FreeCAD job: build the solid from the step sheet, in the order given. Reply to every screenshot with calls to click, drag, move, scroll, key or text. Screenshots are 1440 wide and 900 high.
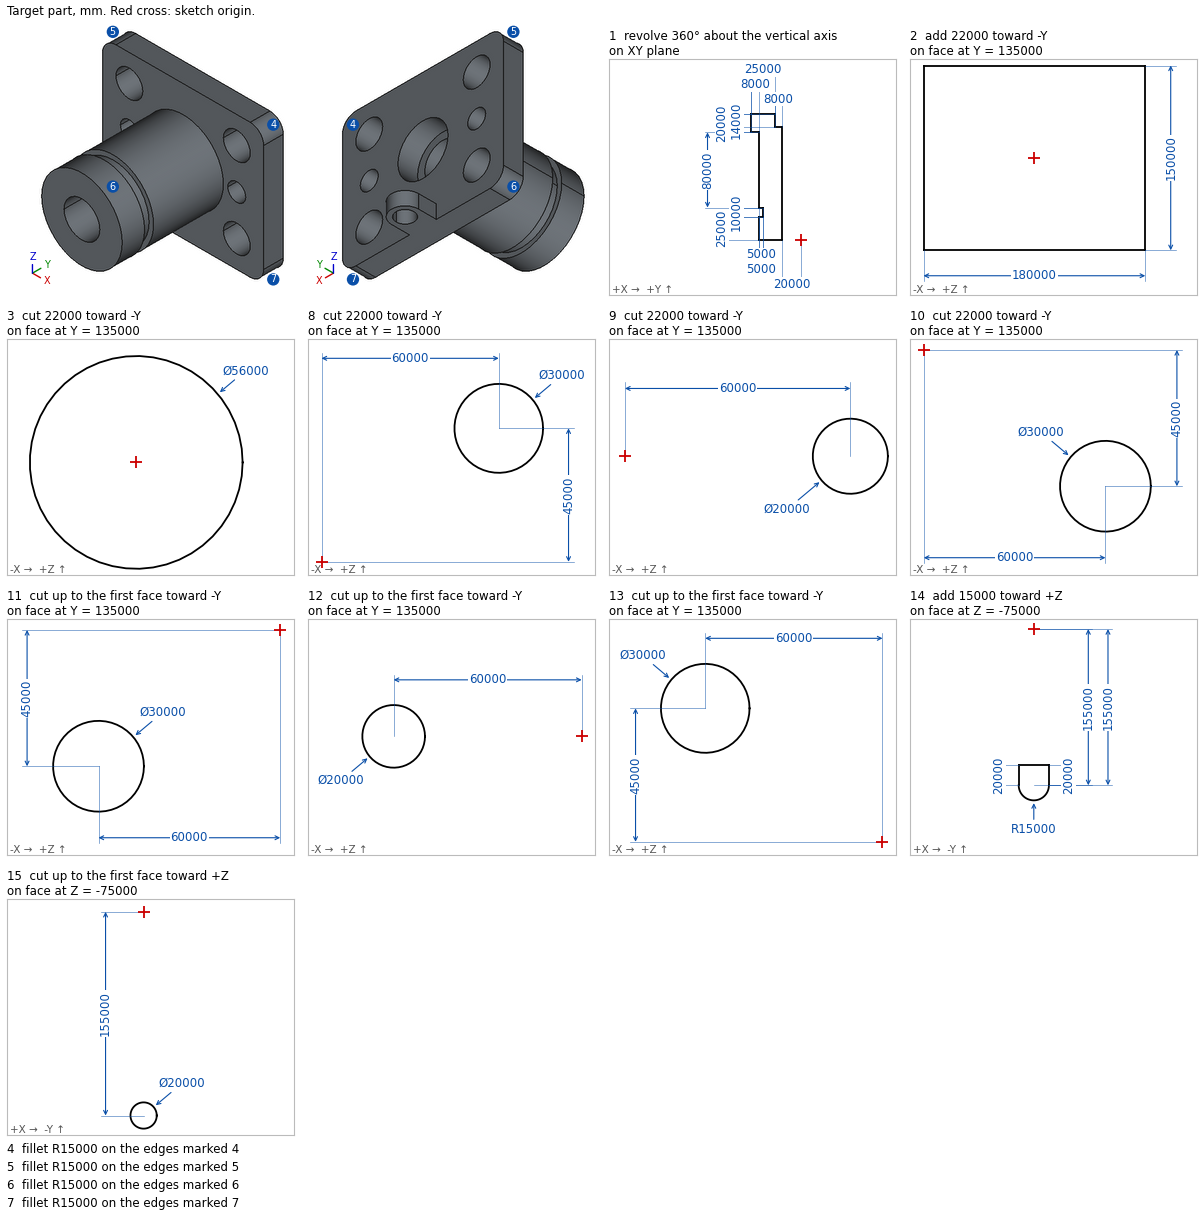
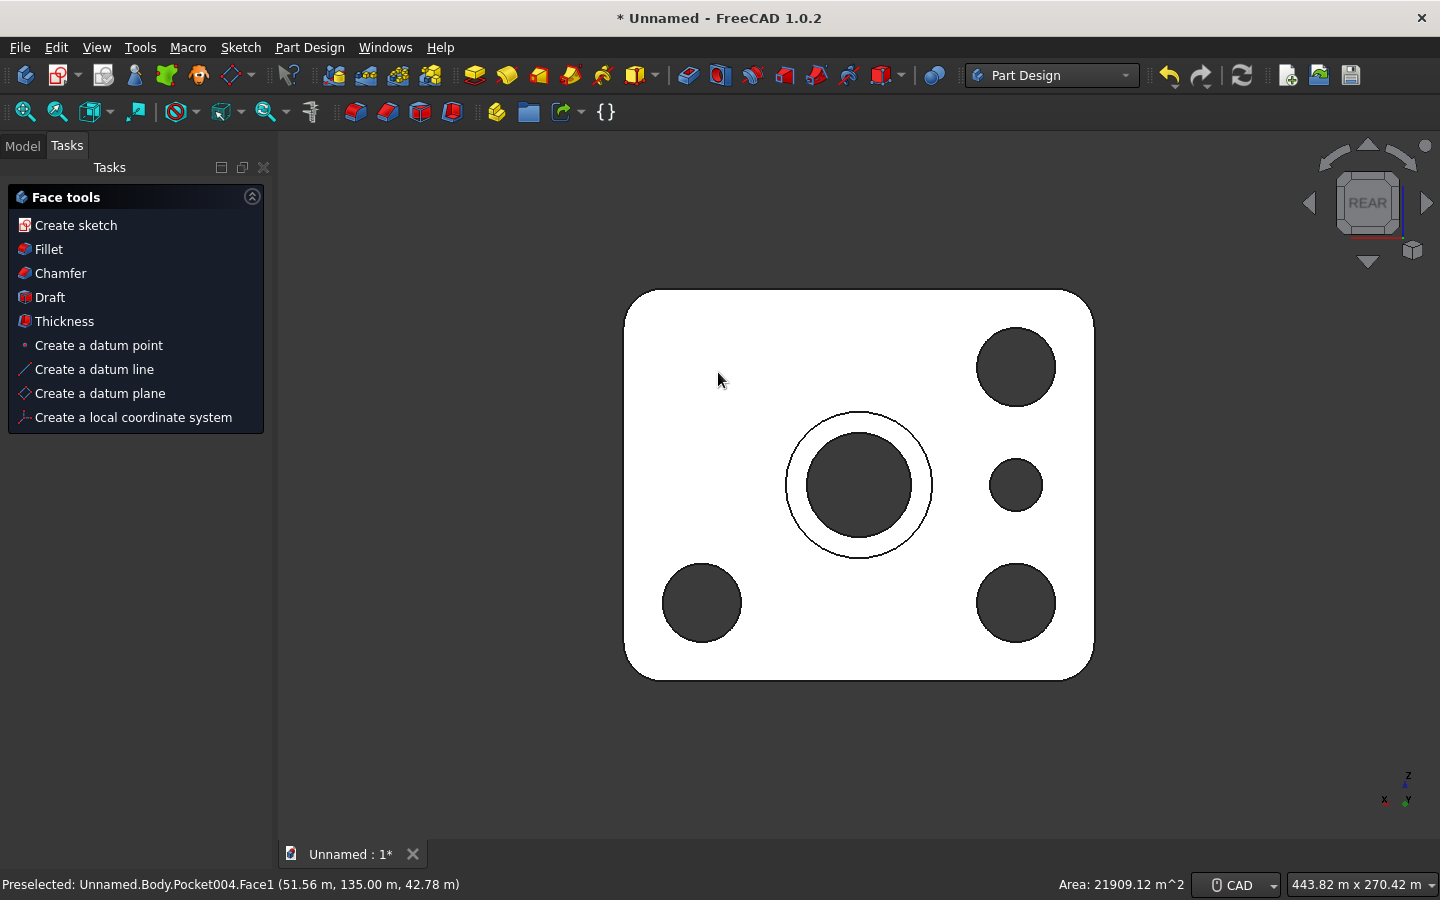
click(58, 76)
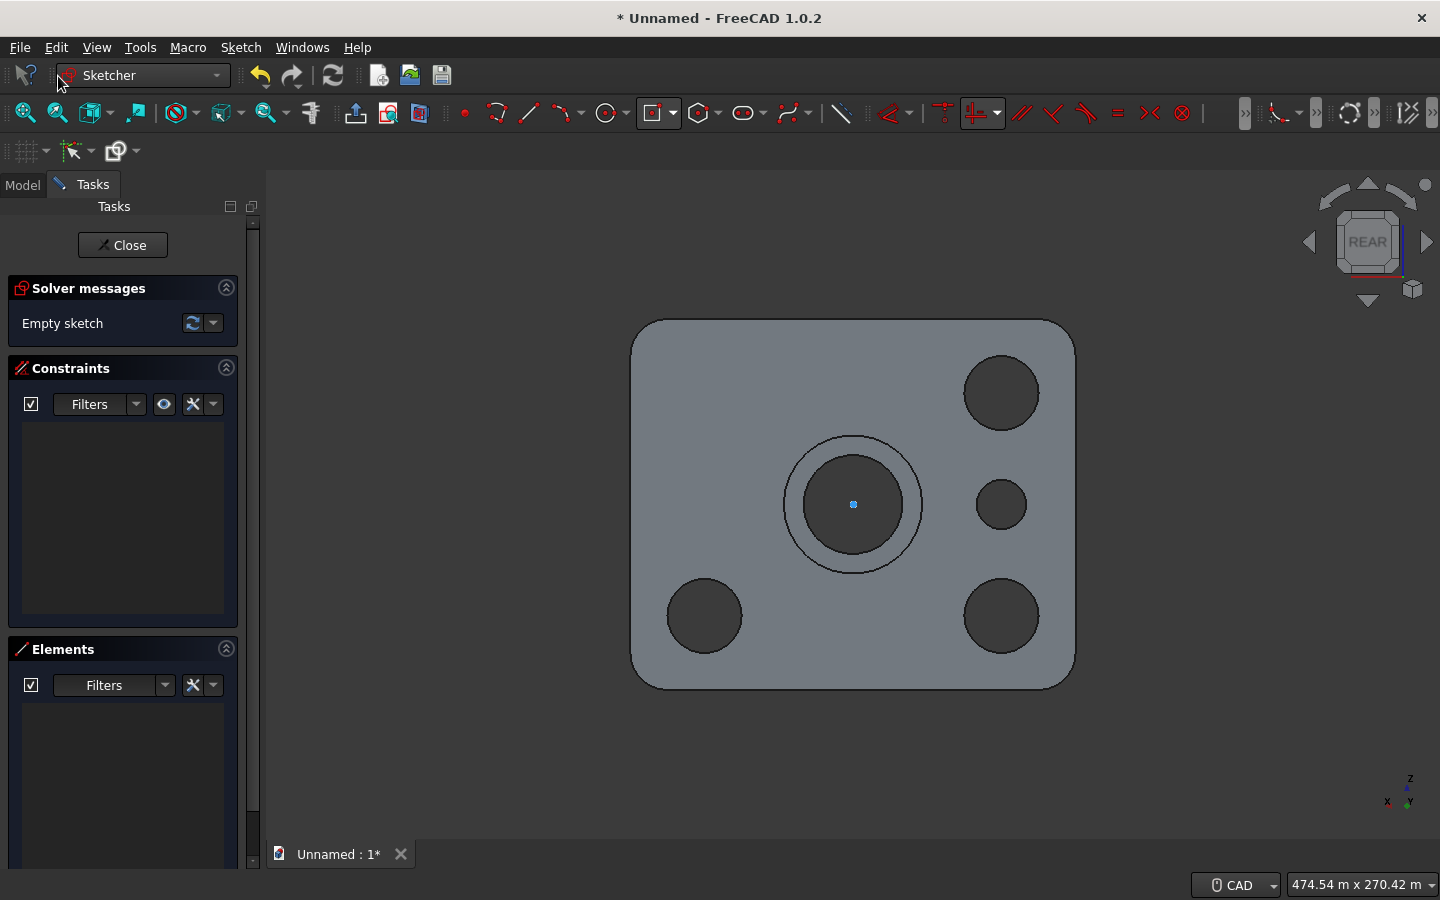
scroll(695, 504, up, 11)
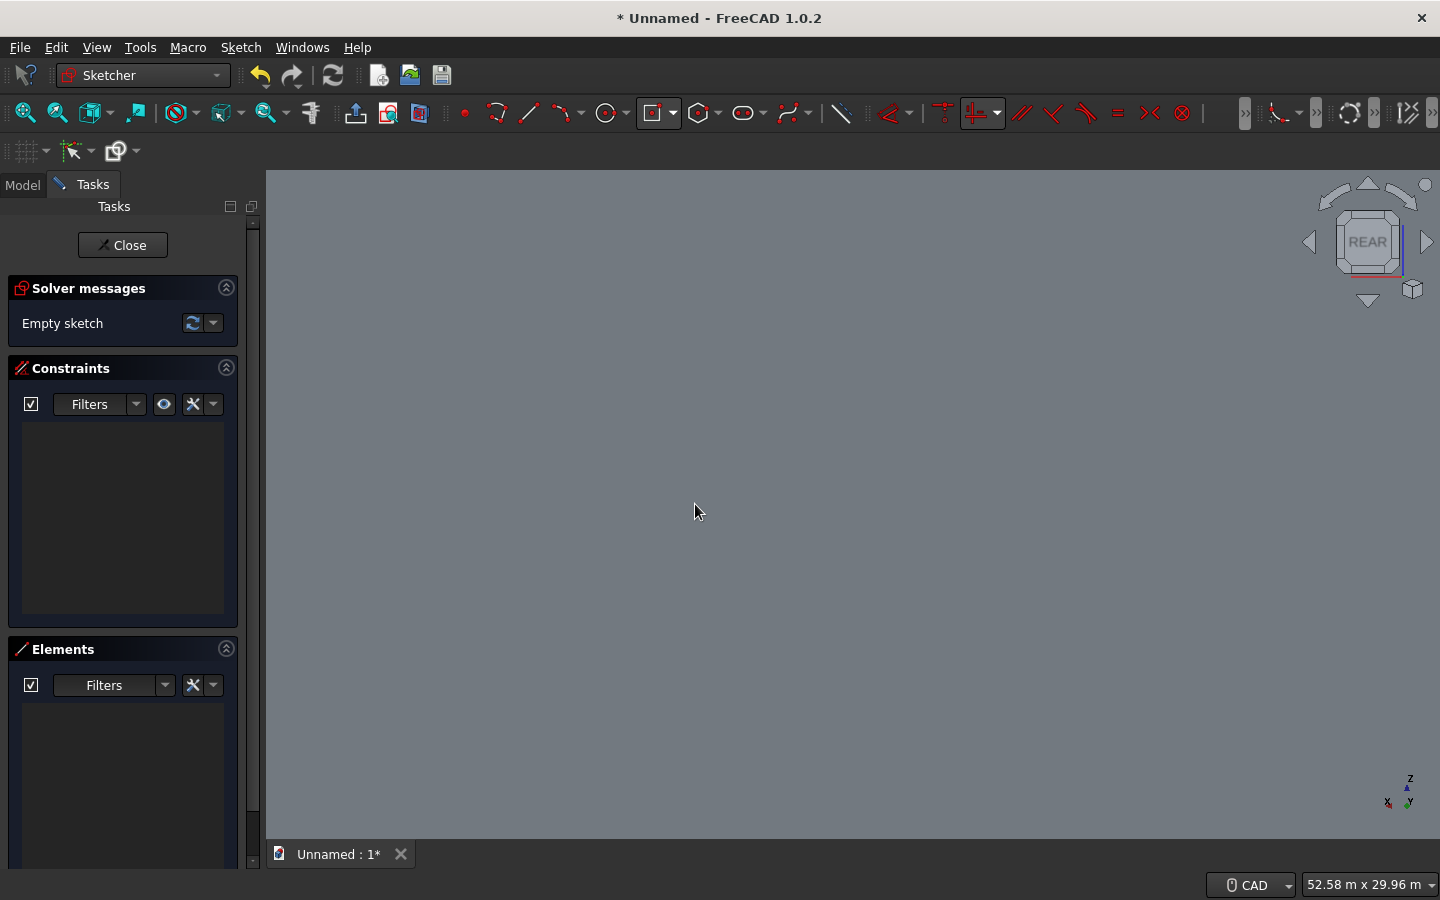
key(g)
key(c)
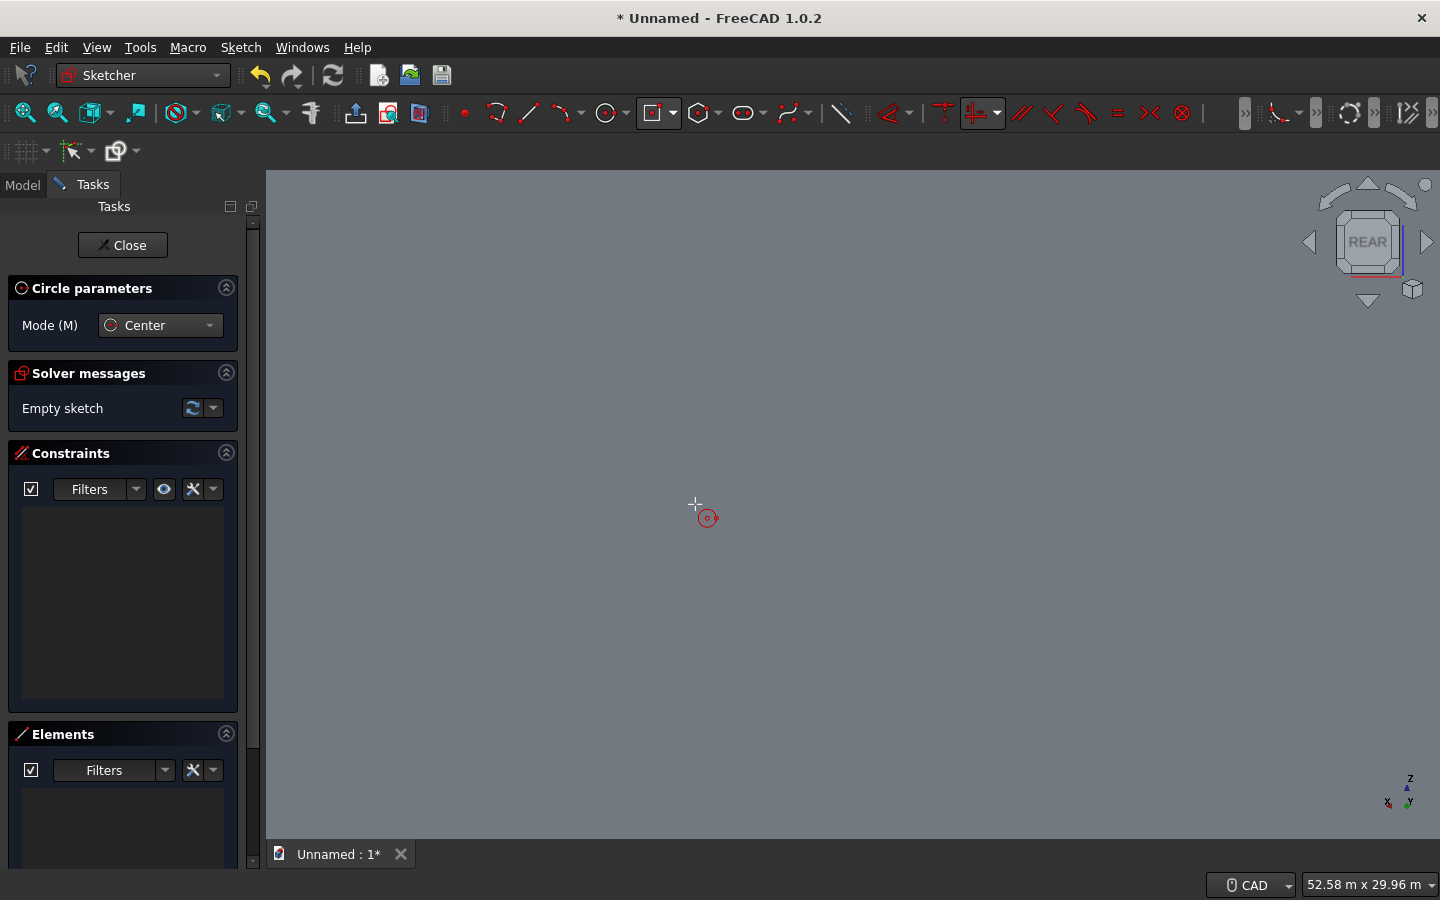
click(778, 504)
click(936, 347)
key(Escape)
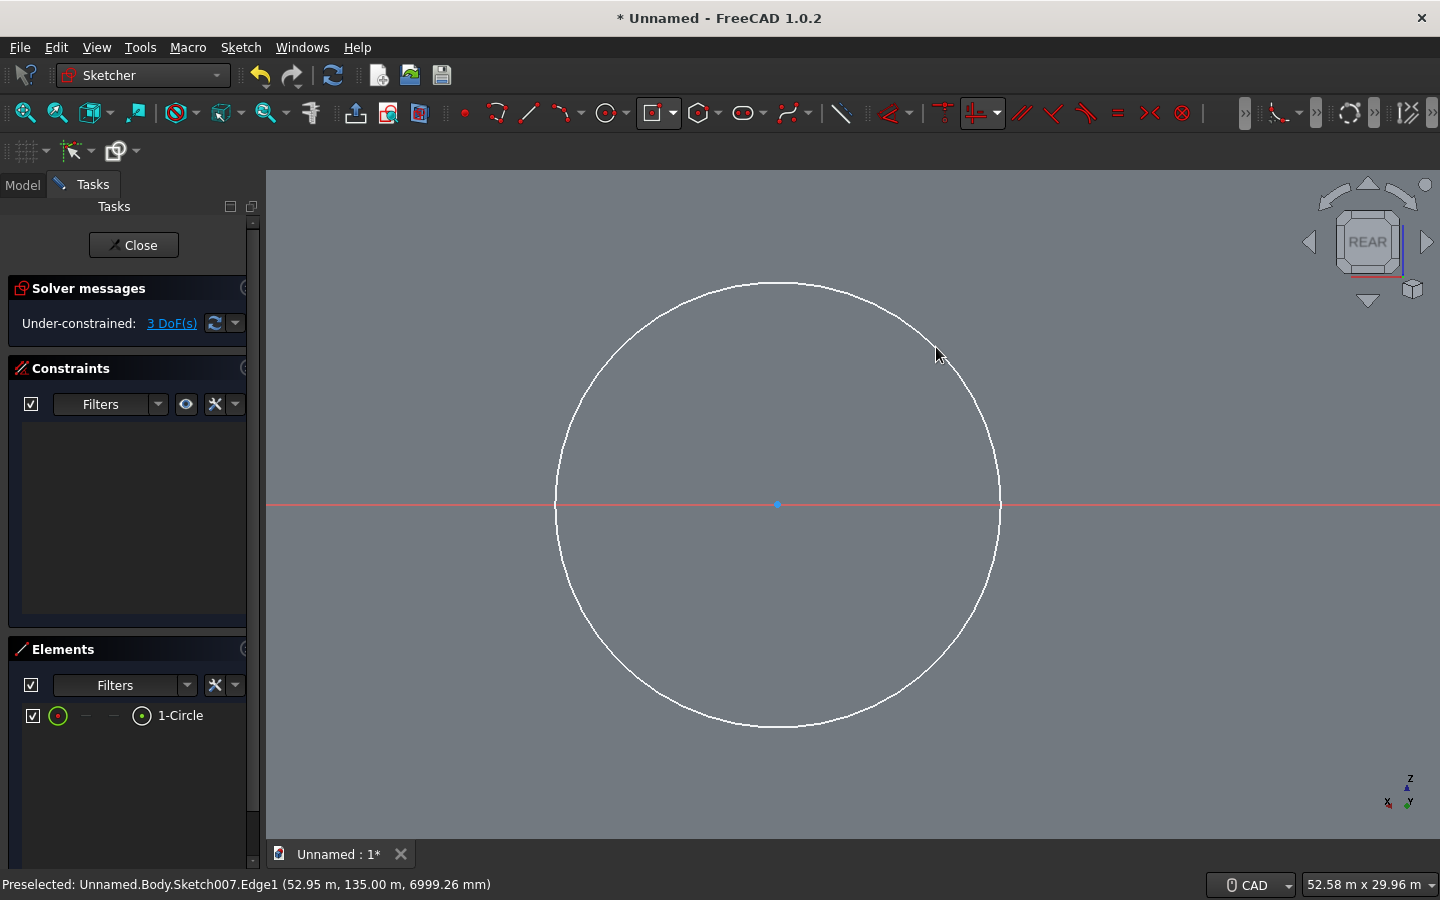
click(778, 505)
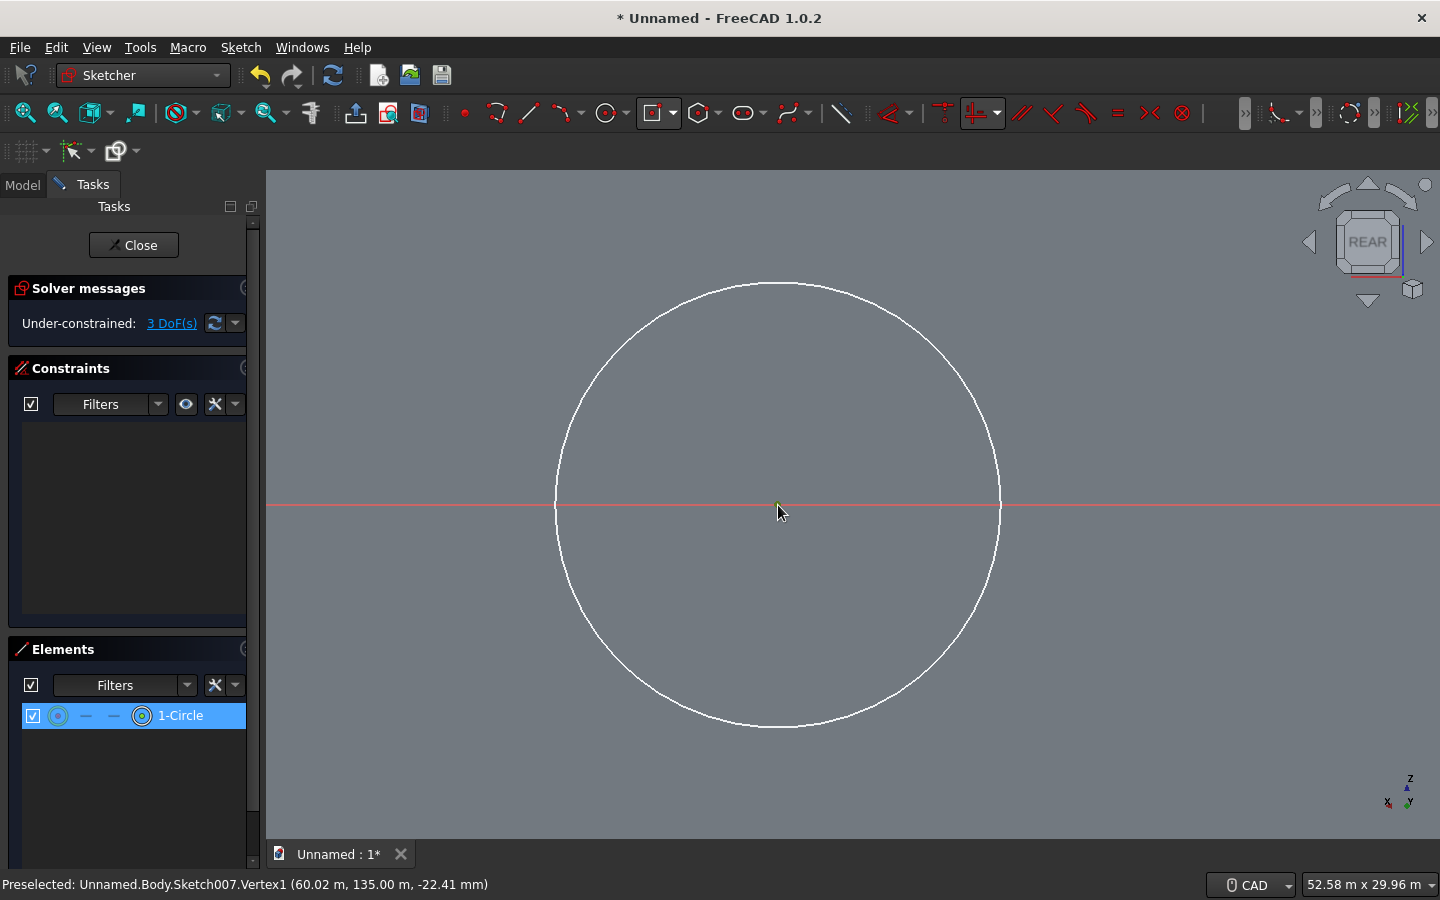
click(364, 504)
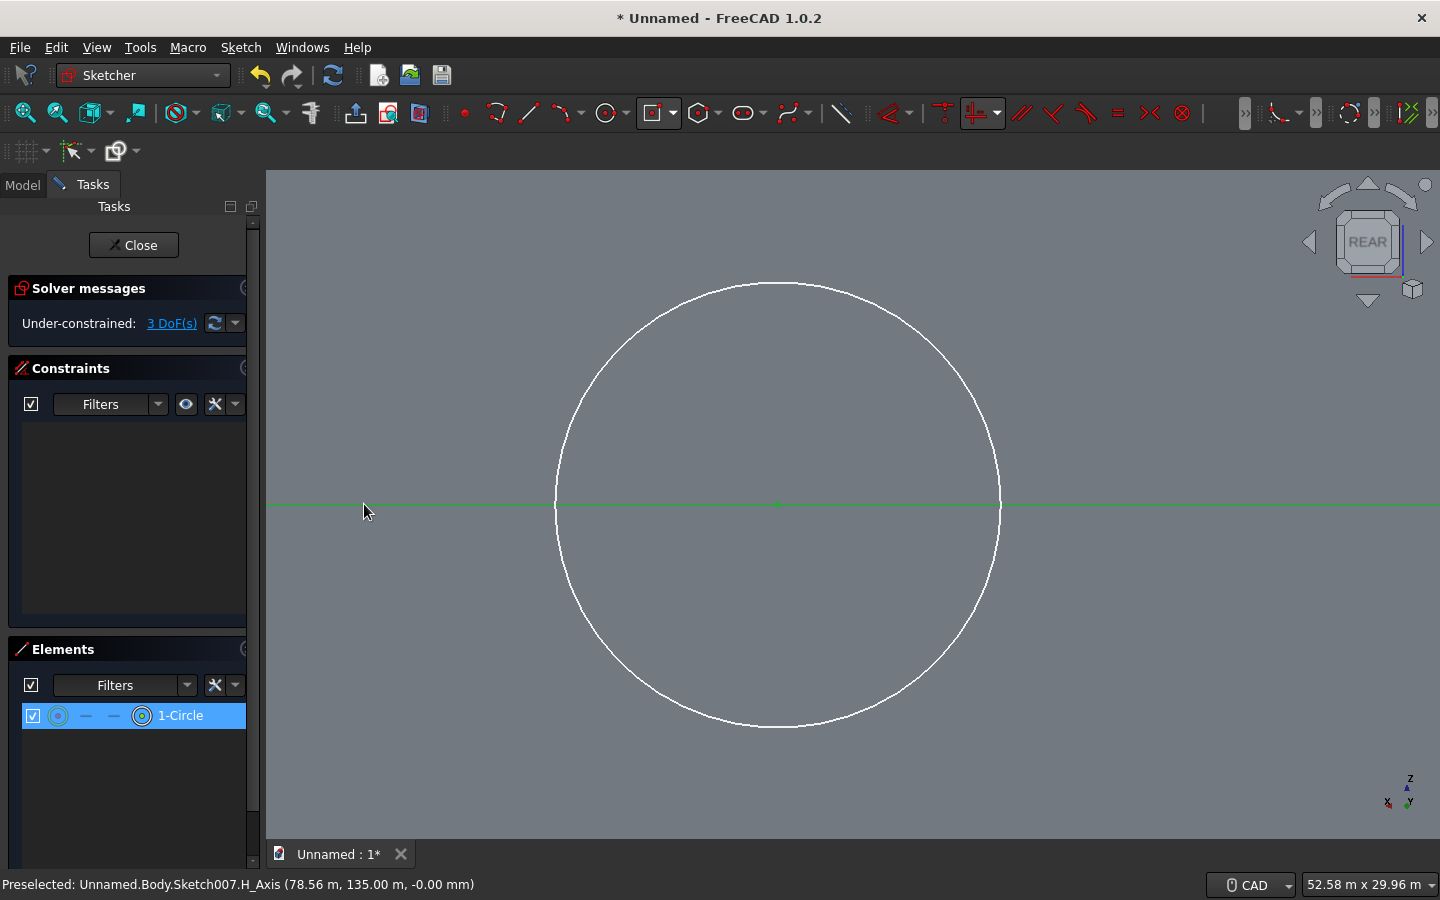
key(c)